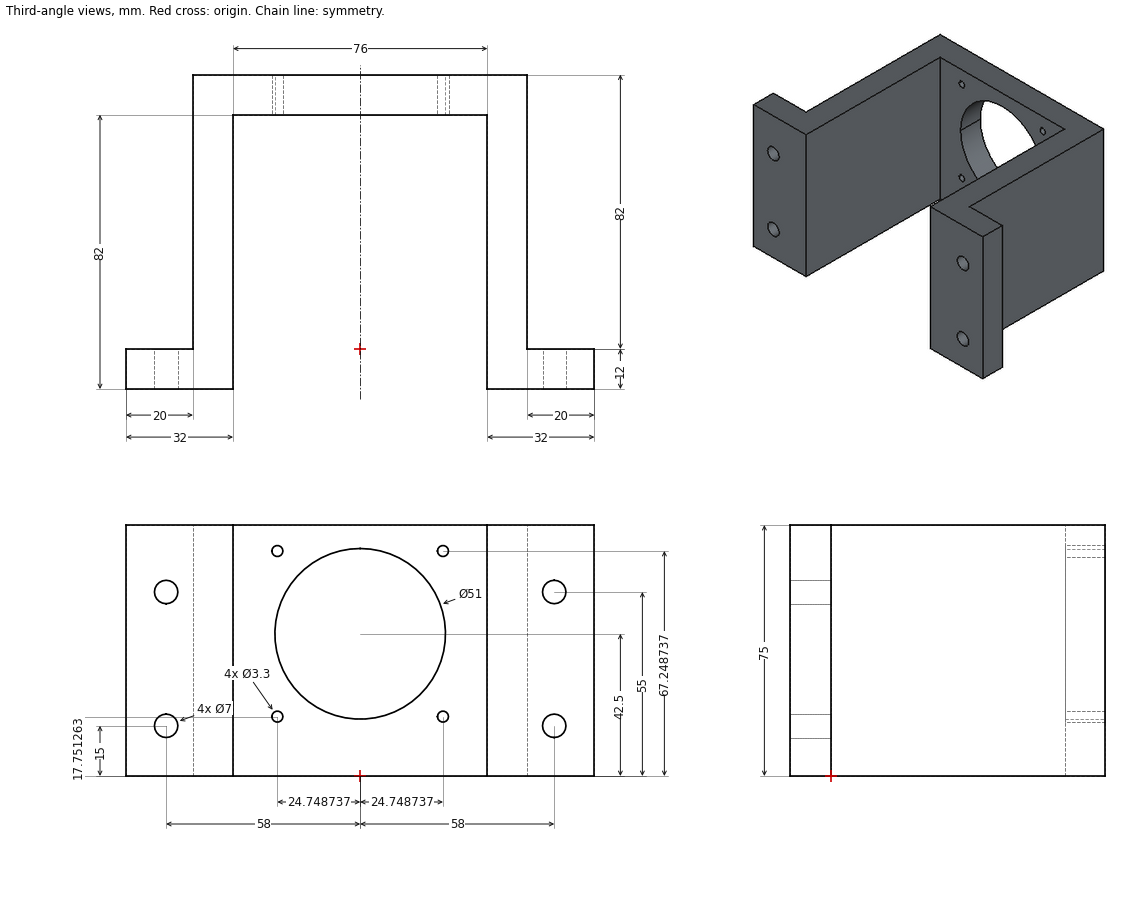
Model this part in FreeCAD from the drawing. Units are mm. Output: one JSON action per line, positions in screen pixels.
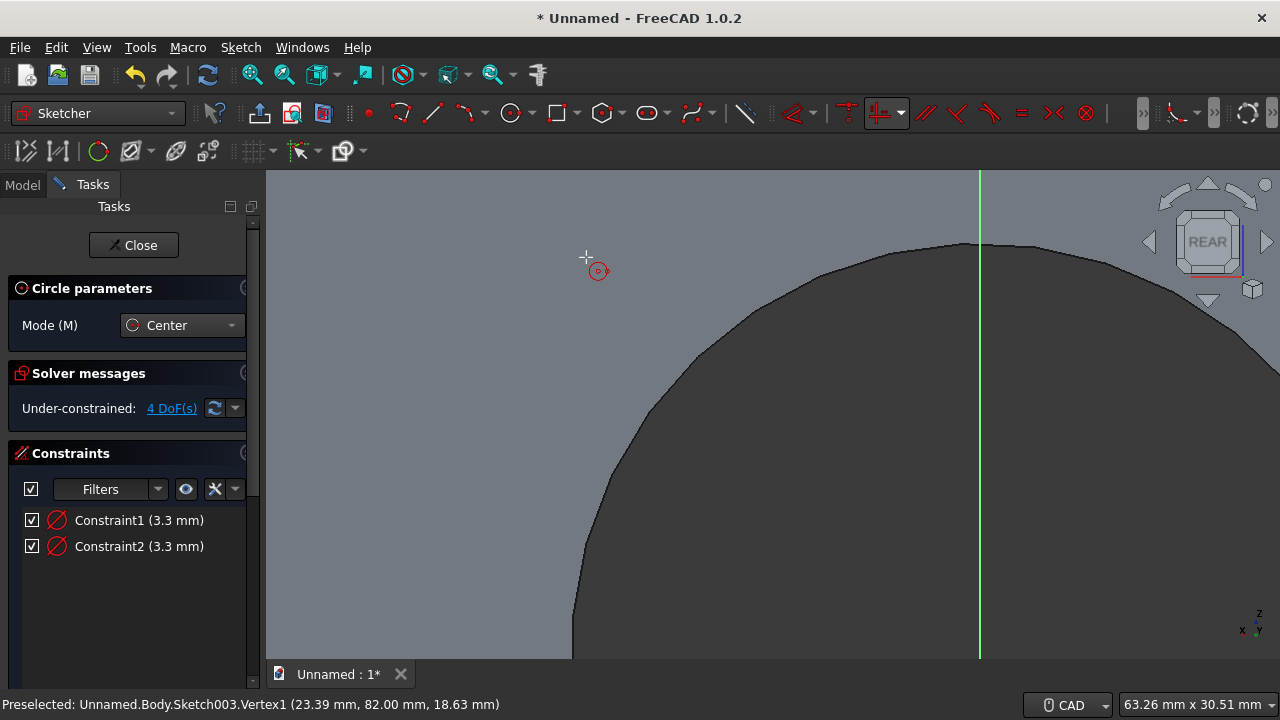
{"action": "left_click", "coordinate": [584, 256]}
{"action": "mouse_move", "coordinate": [602, 237]}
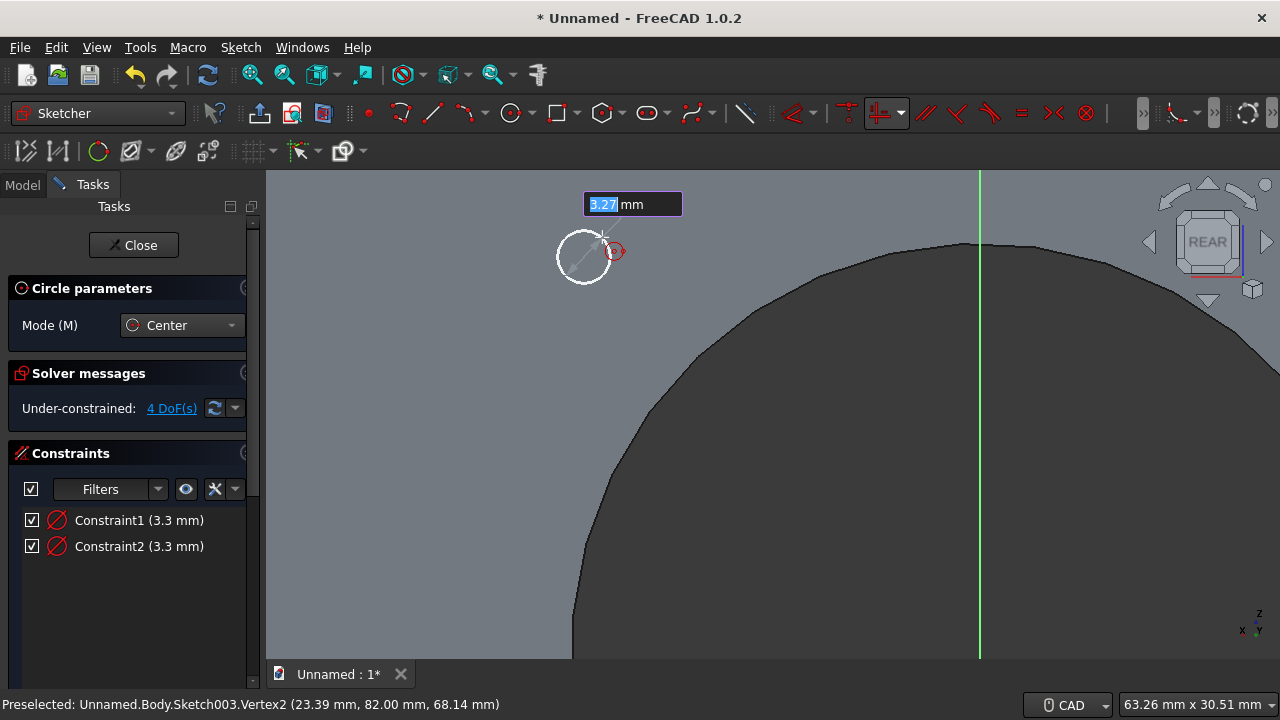
{"action": "type", "text": "3.3"}
{"action": "key", "text": "Return"}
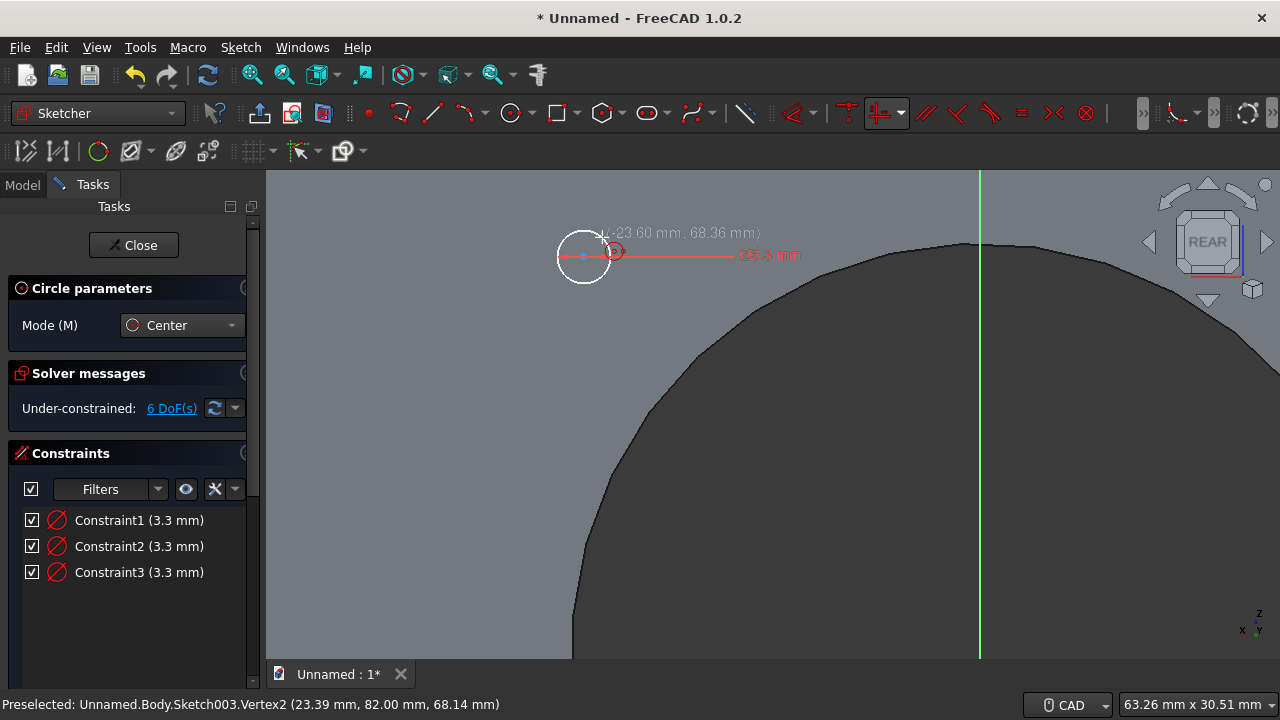
{"action": "scroll", "coordinate": [586, 256], "scroll_direction": "down", "scroll_amount": 6}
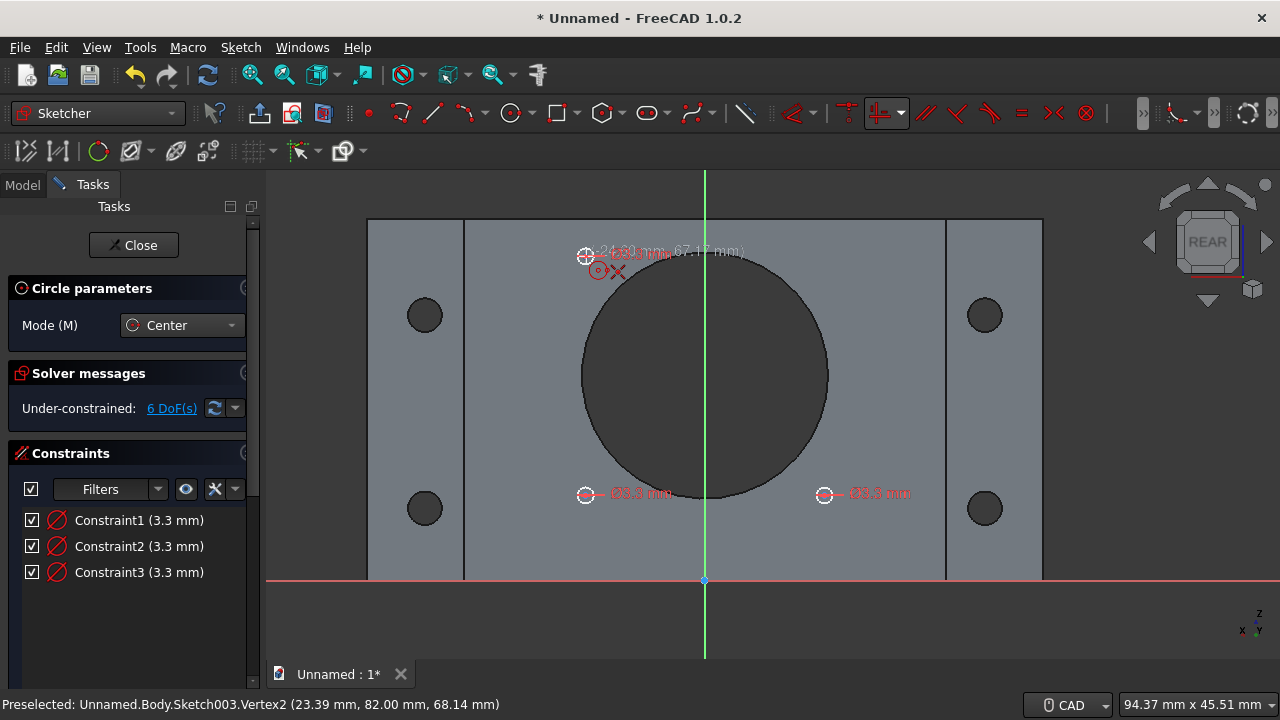
{"action": "scroll", "coordinate": [824, 256], "scroll_direction": "up", "scroll_amount": 6}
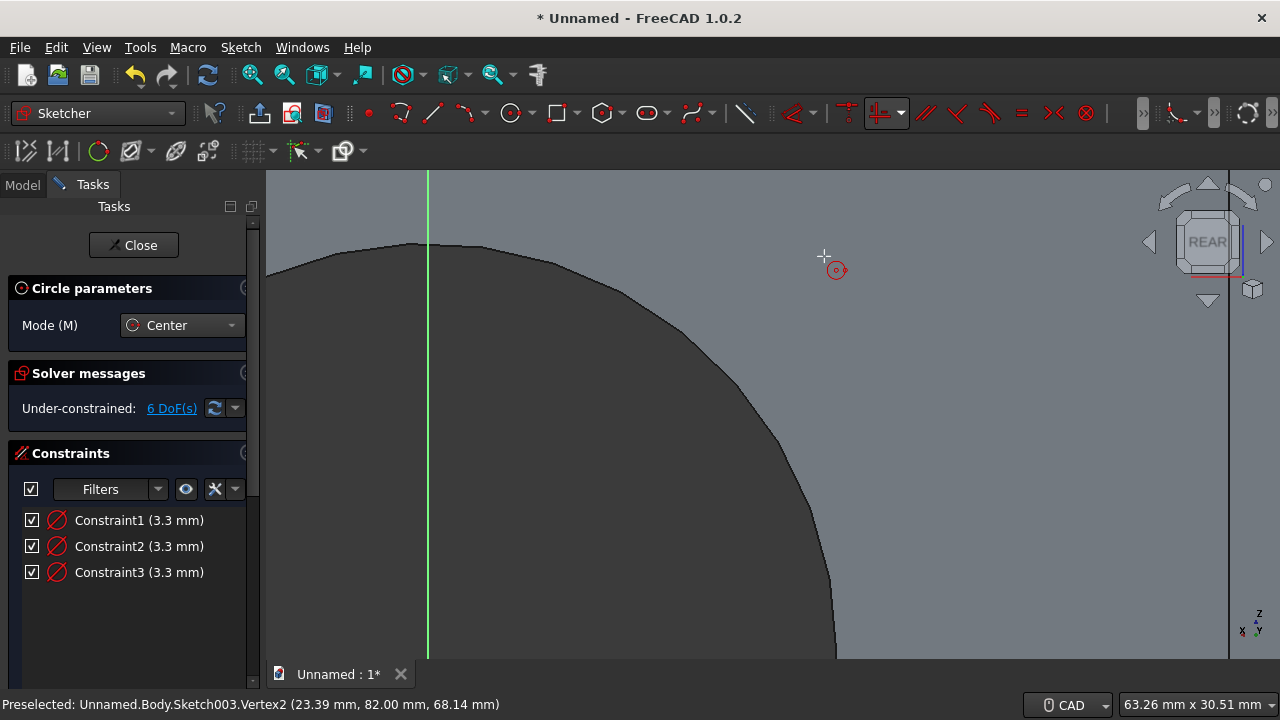
{"action": "left_click", "coordinate": [824, 256]}
{"action": "mouse_move", "coordinate": [843, 237]}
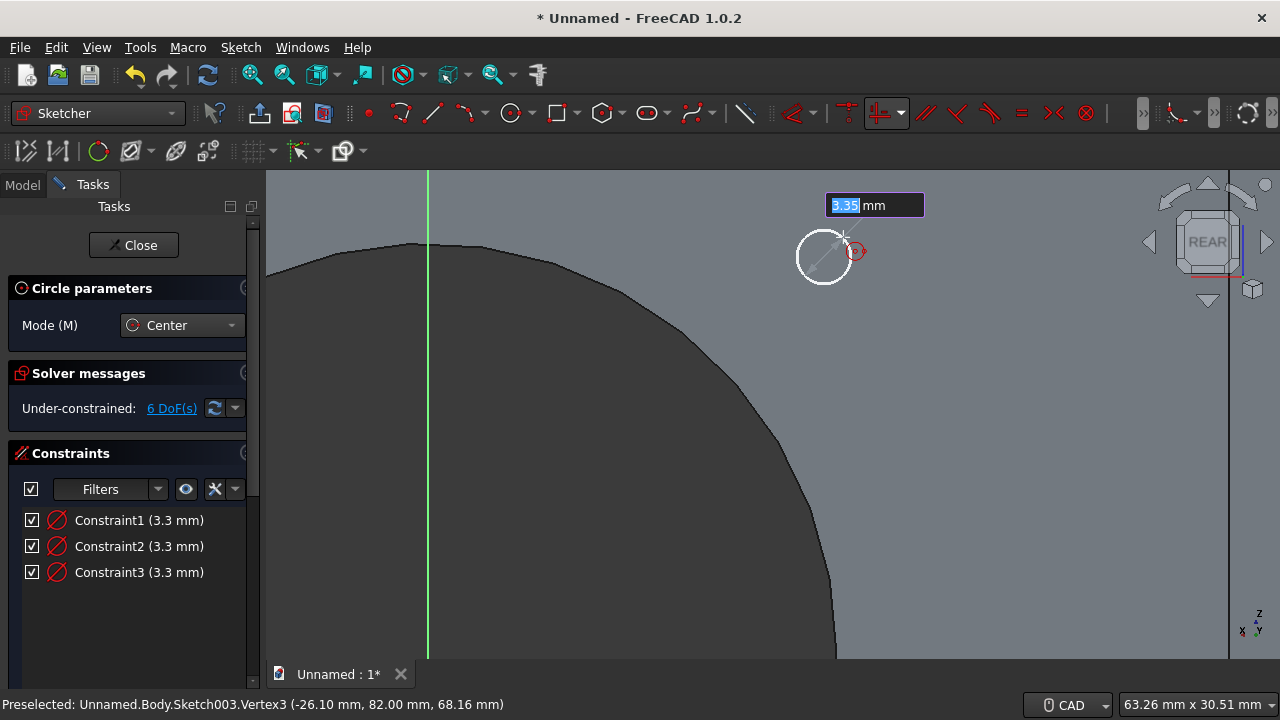
{"action": "type", "text": "3.3"}
{"action": "key", "text": "Return"}
{"action": "key", "text": "Escape"}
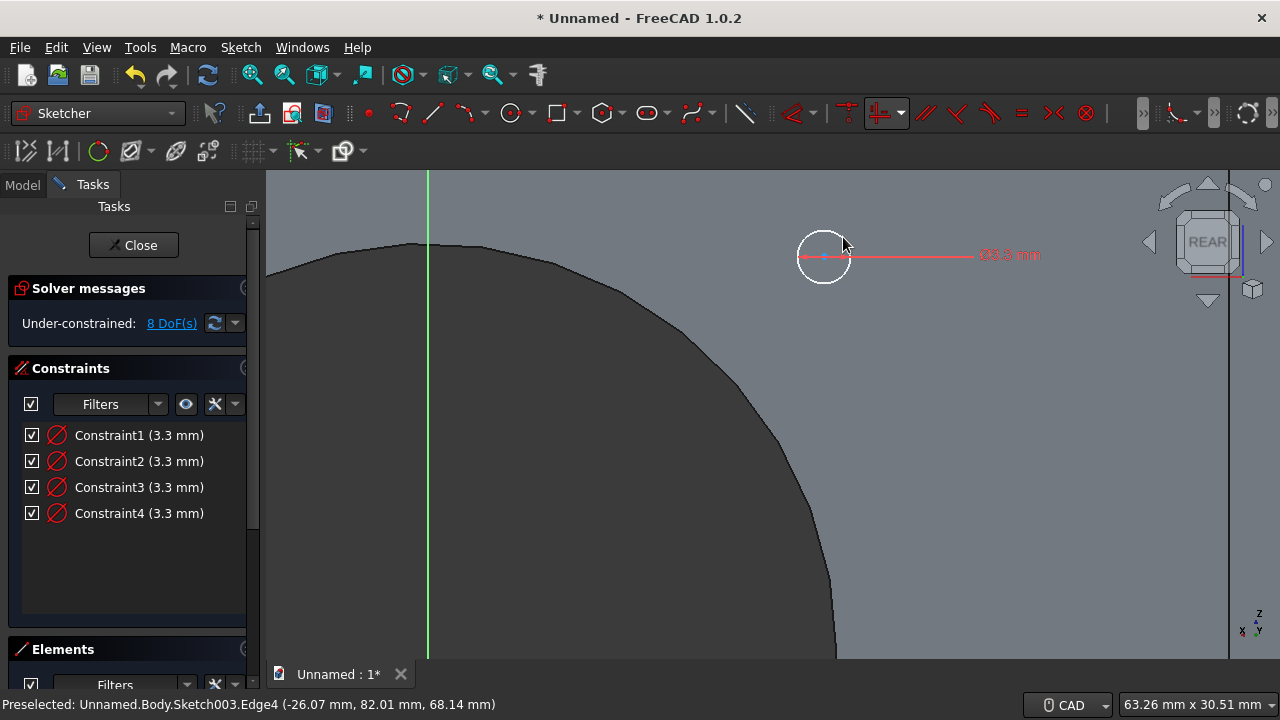
{"action": "scroll", "coordinate": [824, 256], "scroll_direction": "down", "scroll_amount": 6}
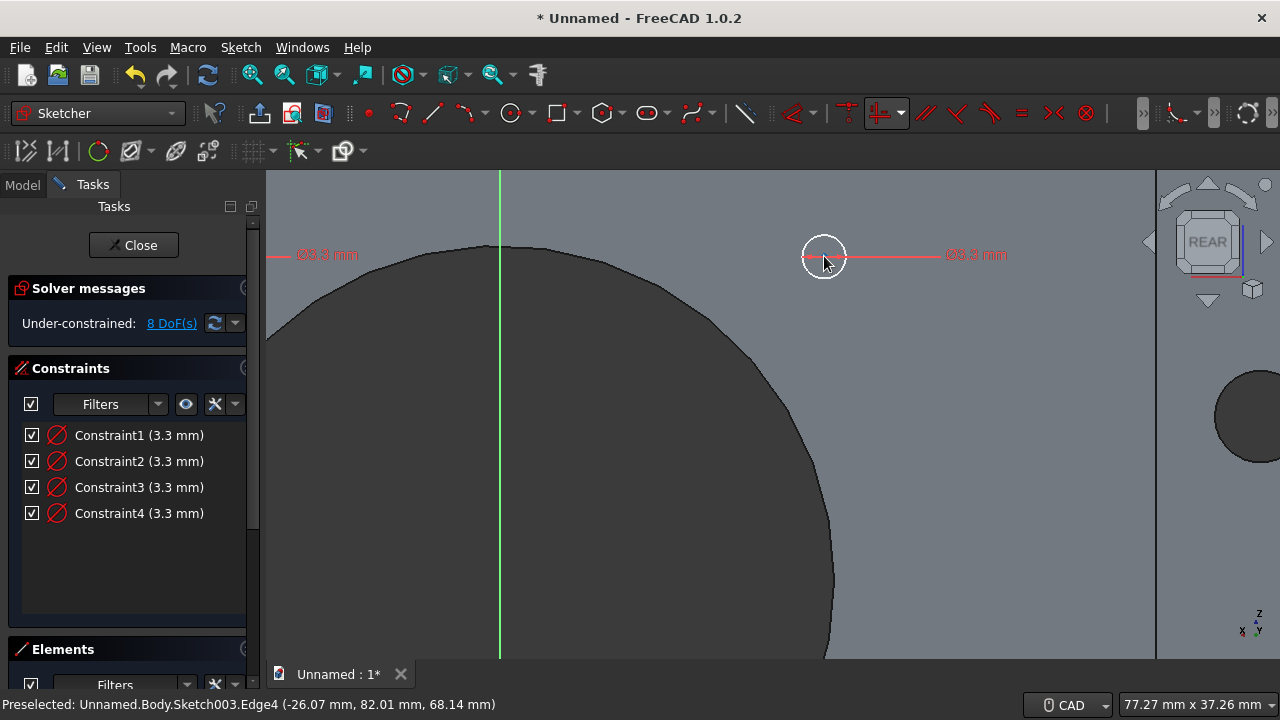
{"action": "left_click", "coordinate": [824, 495]}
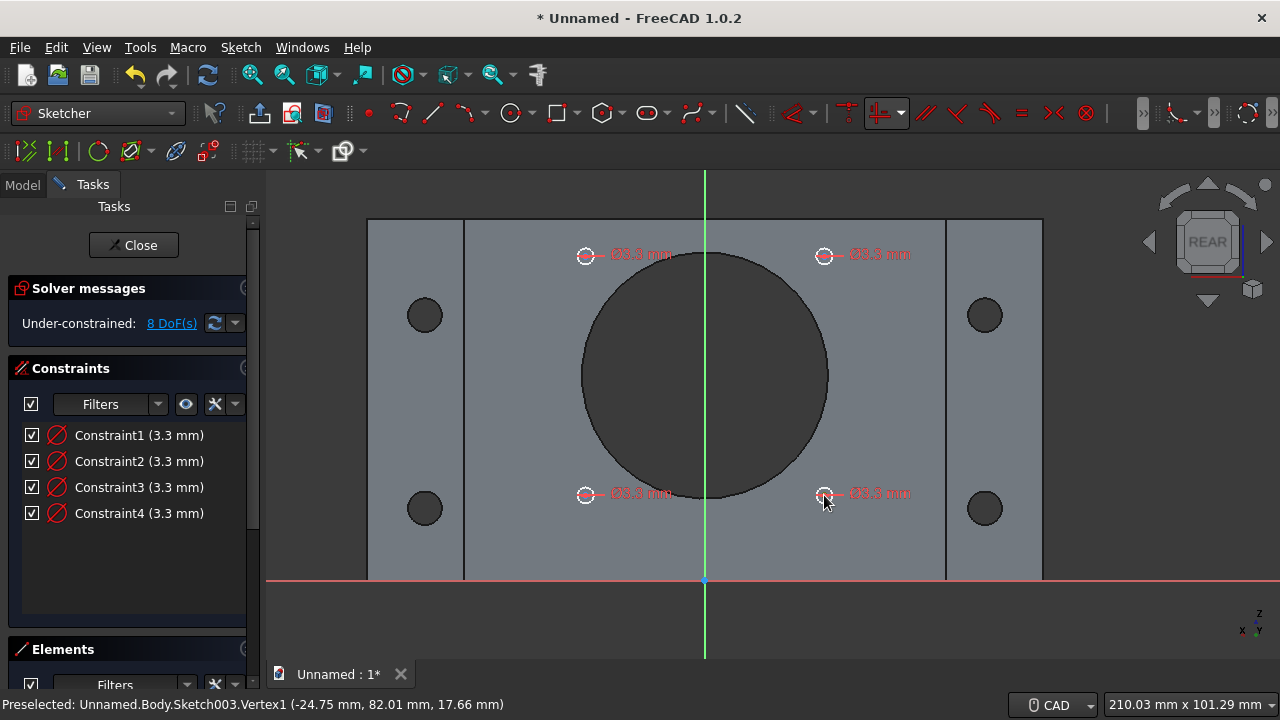
{"action": "left_click", "coordinate": [586, 495]}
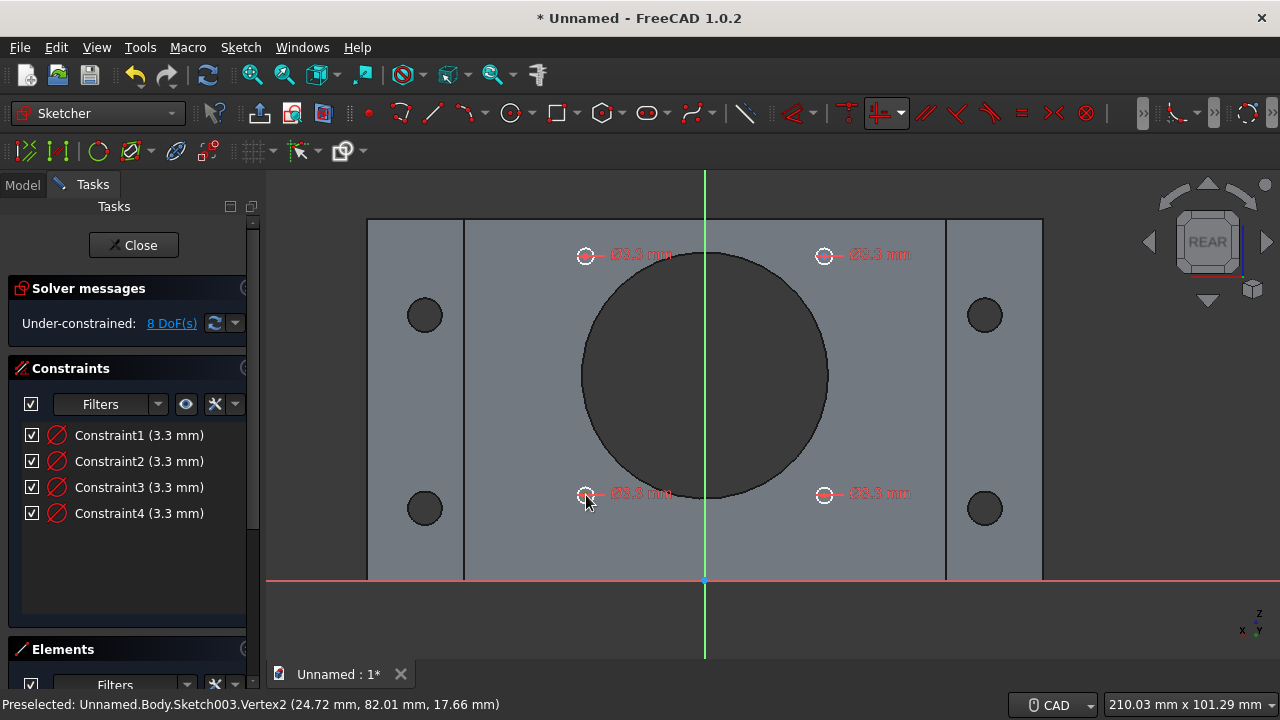
{"action": "key", "text": "h"}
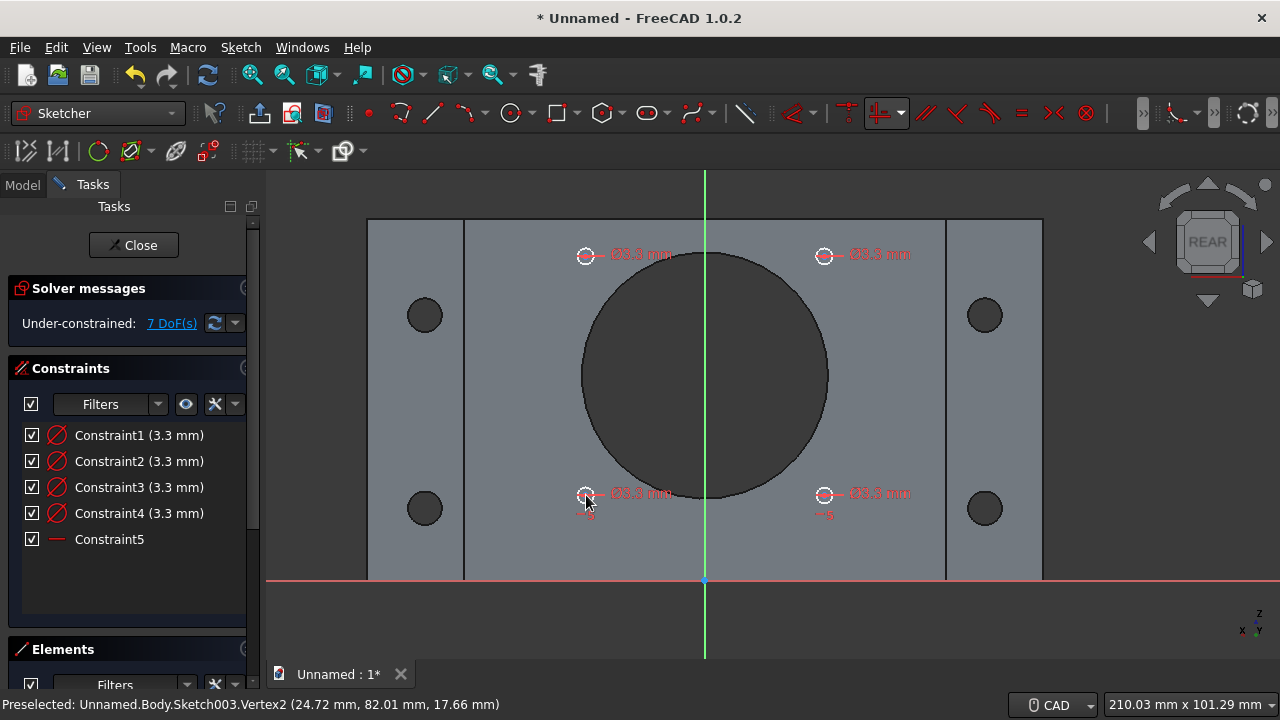
{"action": "left_click", "coordinate": [586, 495]}